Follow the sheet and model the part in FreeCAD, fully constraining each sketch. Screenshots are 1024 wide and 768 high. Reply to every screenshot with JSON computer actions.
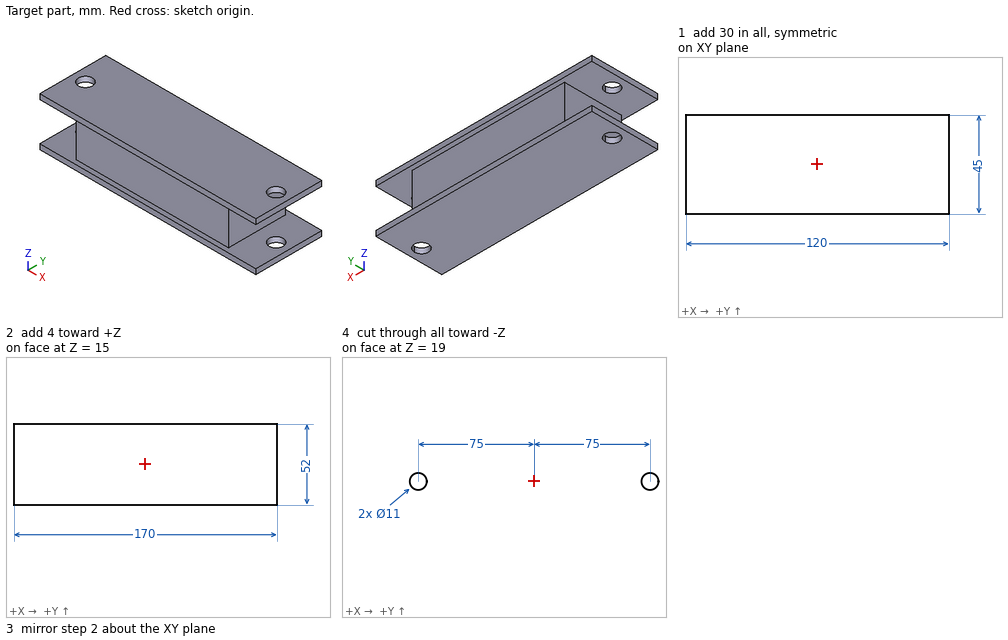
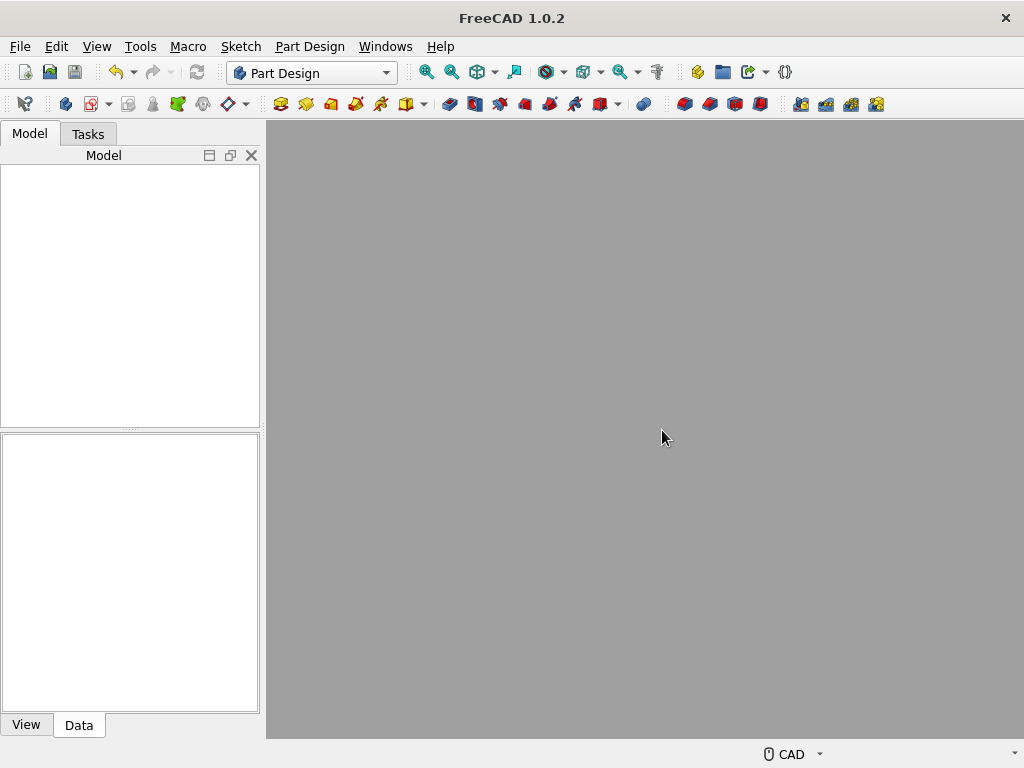
{"action": "left_click", "coordinate": [25, 72]}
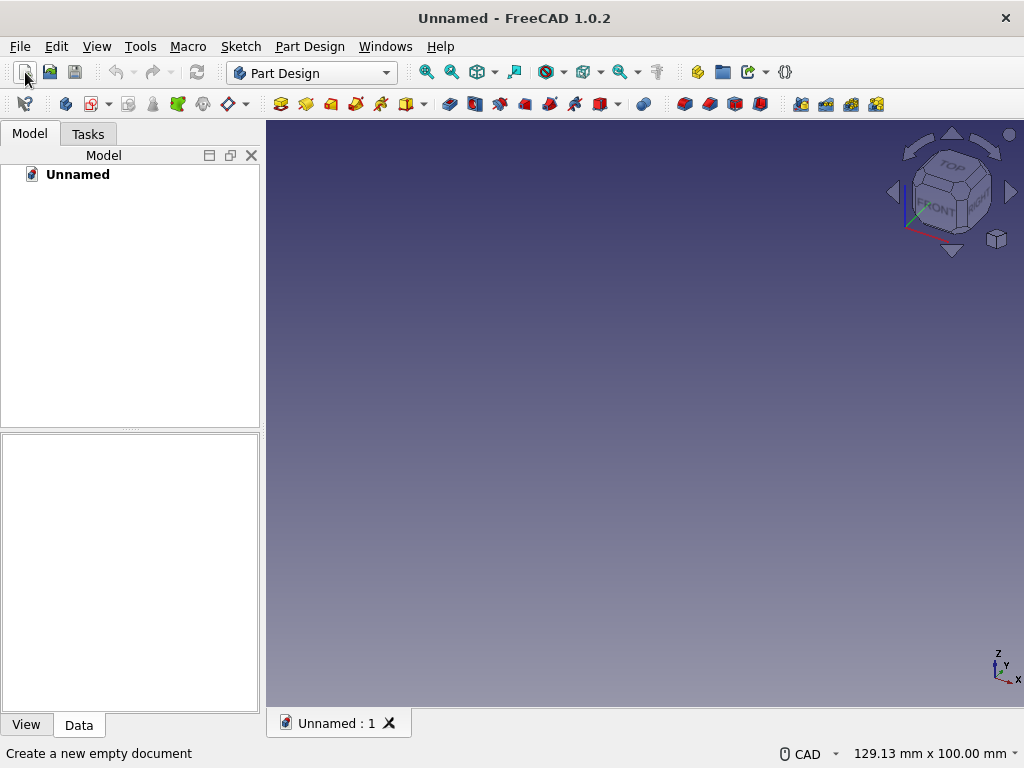
{"action": "left_click", "coordinate": [90, 104]}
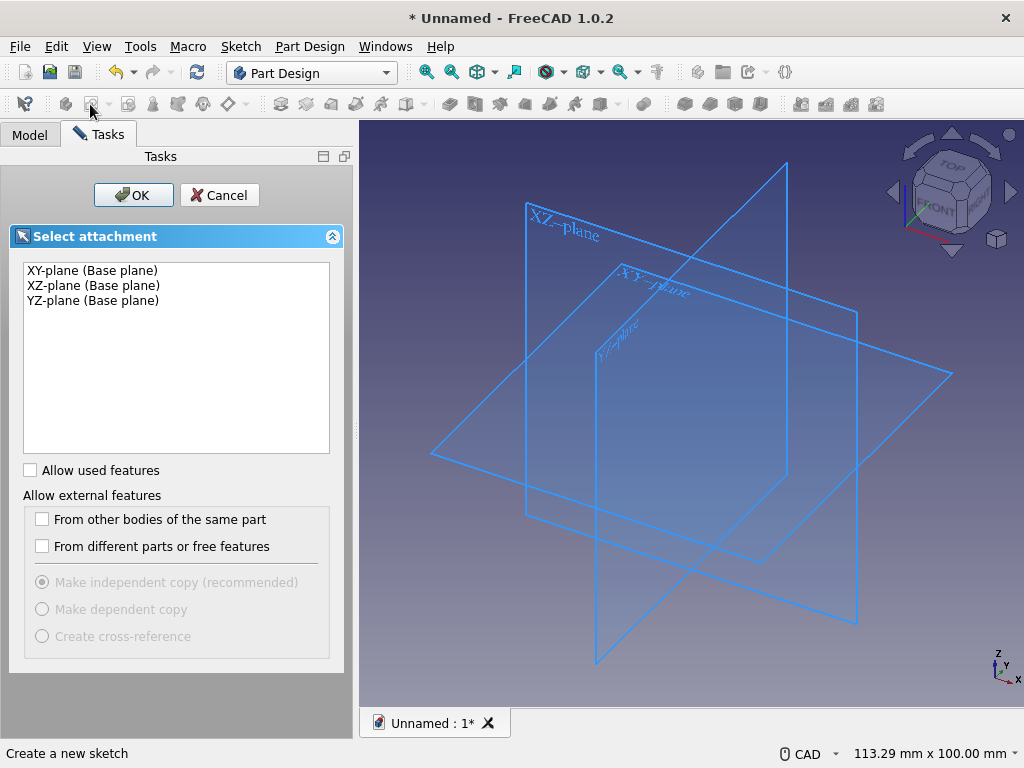
{"action": "left_click", "coordinate": [84, 270]}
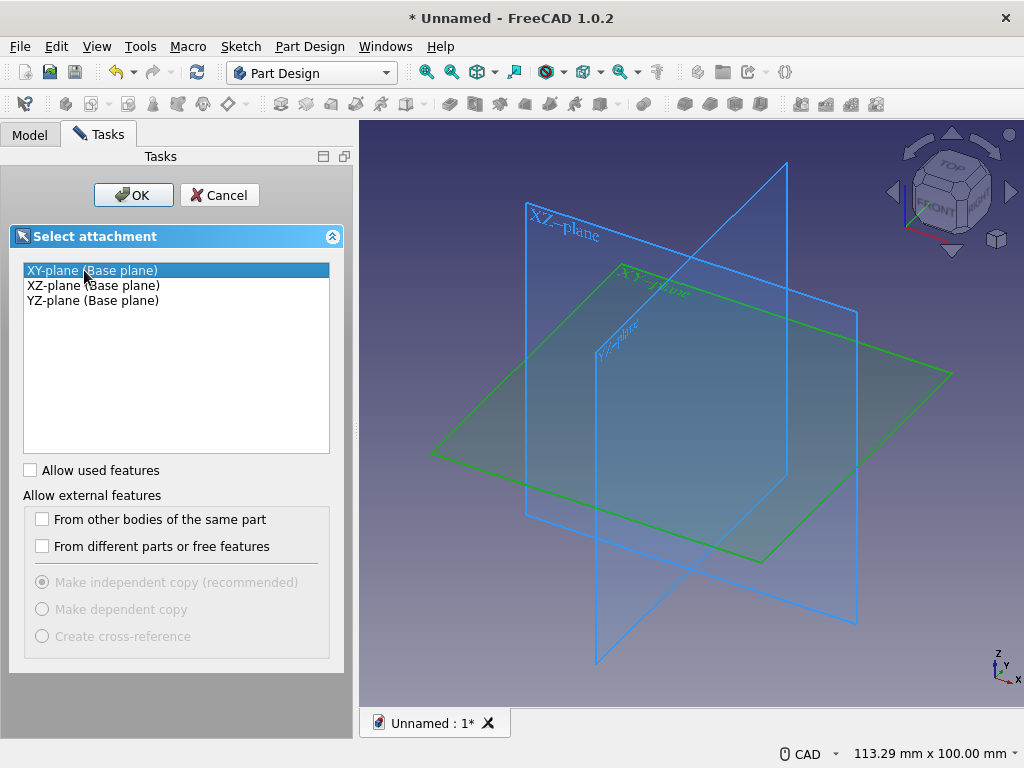
{"action": "left_click", "coordinate": [134, 195]}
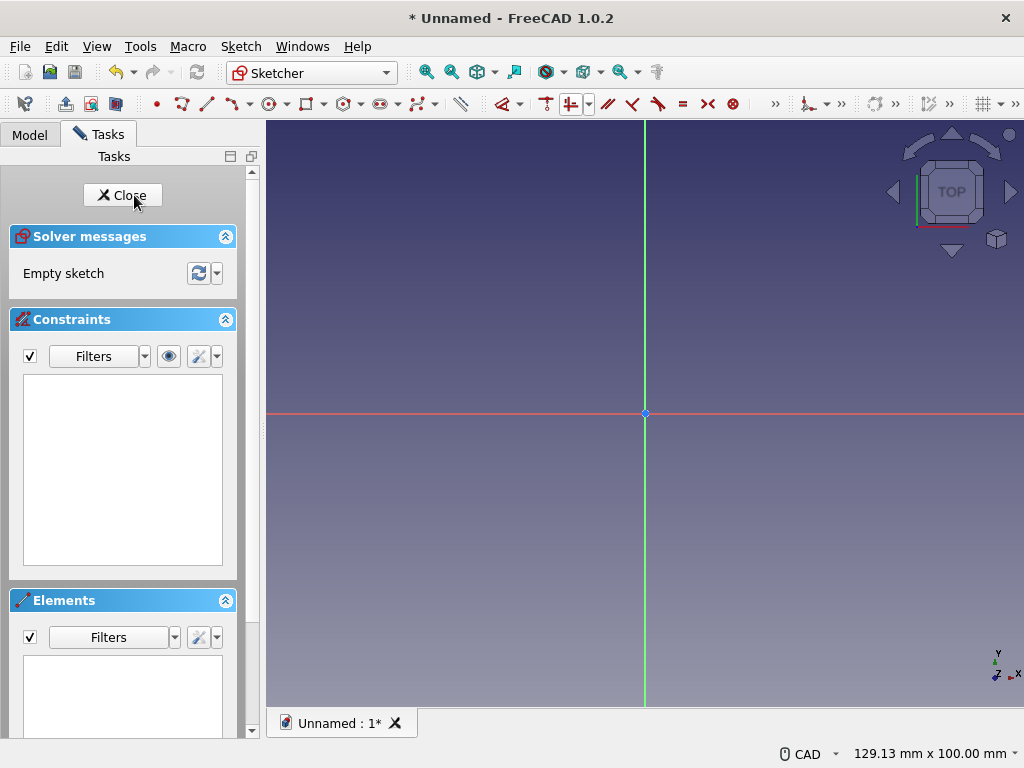
{"action": "scroll", "coordinate": [493, 414], "scroll_direction": "down", "scroll_amount": 3}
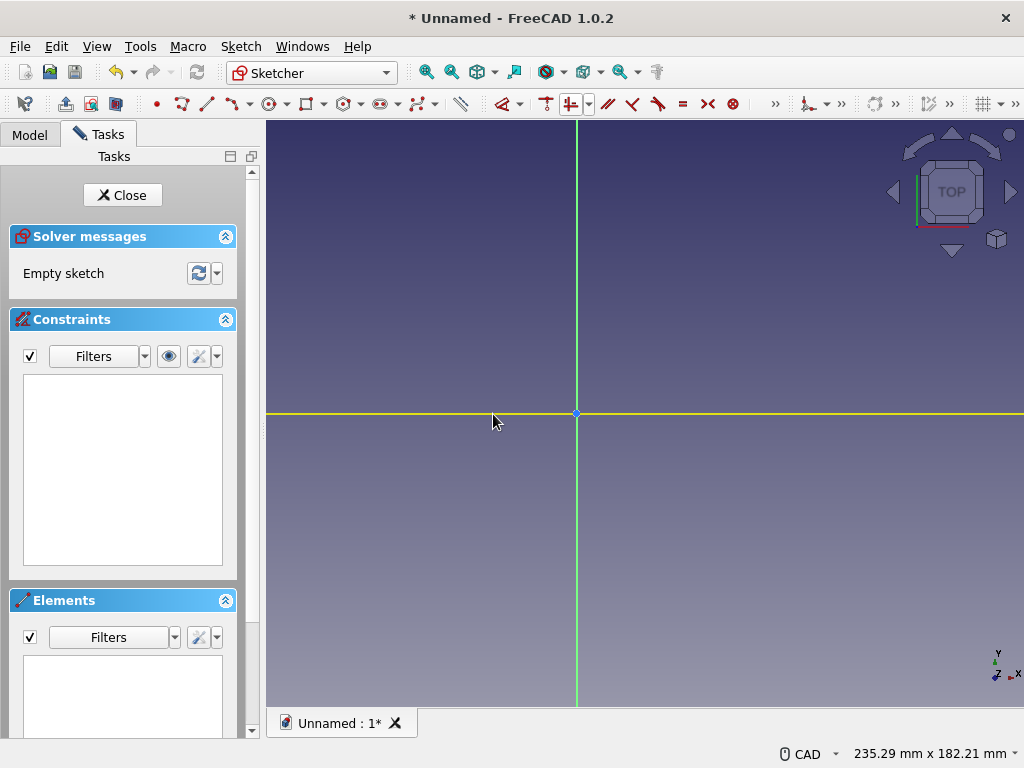
{"action": "left_click", "coordinate": [324, 104]}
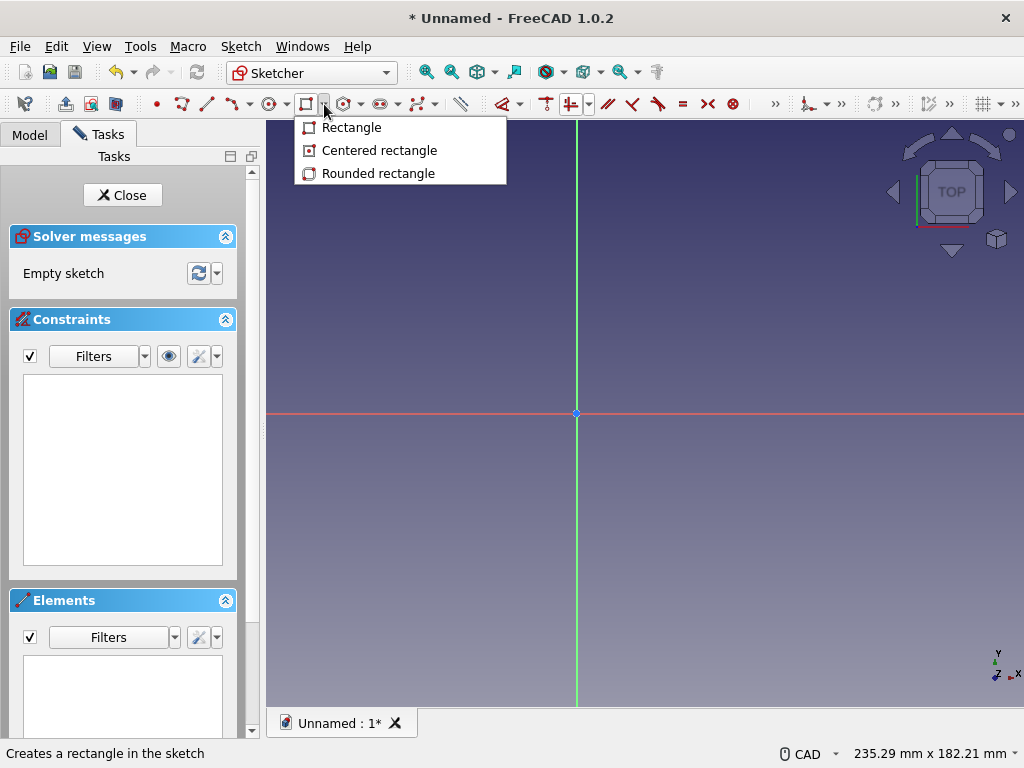
{"action": "left_click", "coordinate": [400, 150]}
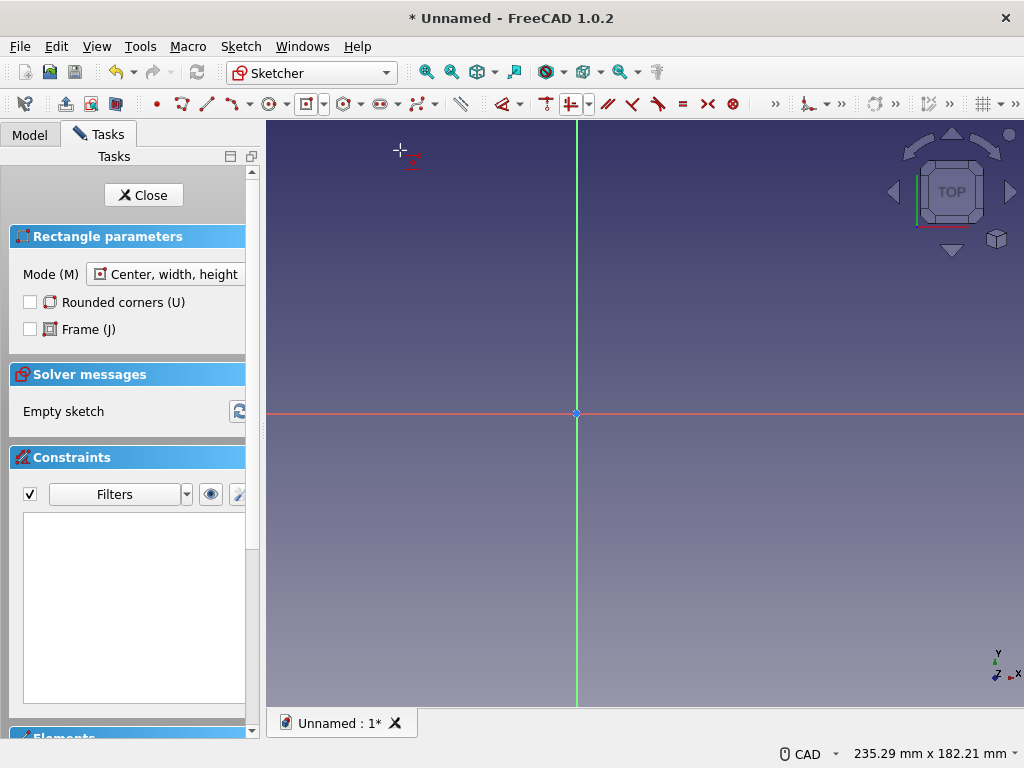
{"action": "left_click", "coordinate": [577, 414]}
{"action": "mouse_move", "coordinate": [770, 341]}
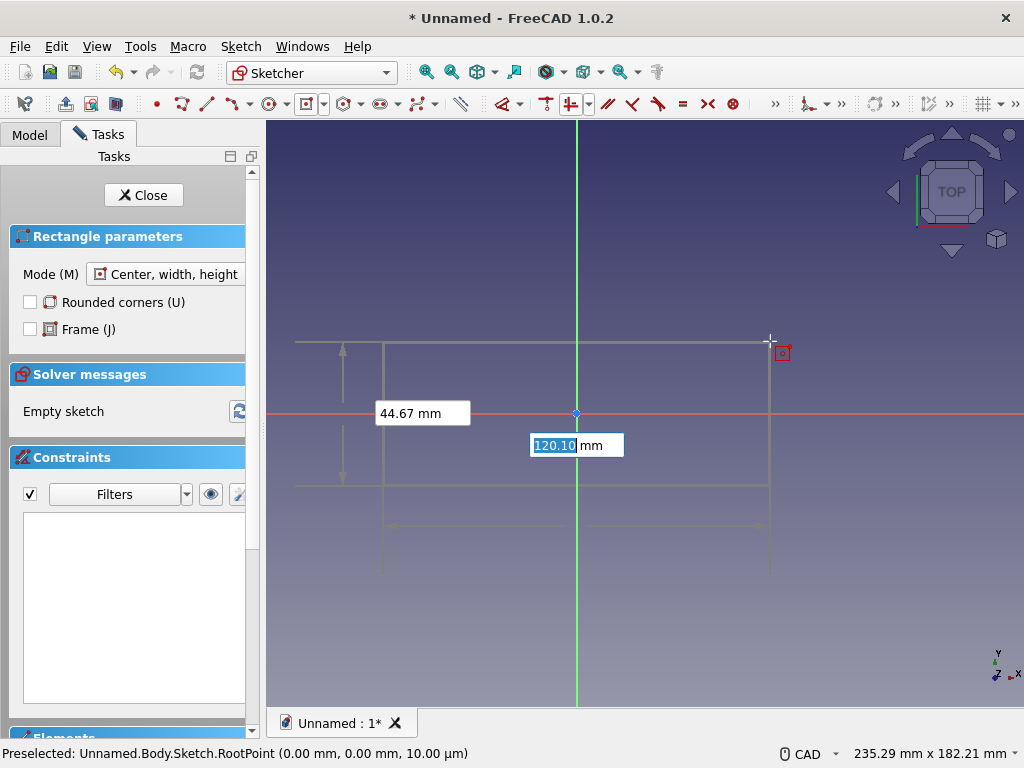
{"action": "type", "text": "120"}
{"action": "key", "text": "Tab"}
{"action": "type", "text": "45"}
{"action": "key", "text": "Return"}
{"action": "key", "text": "Escape"}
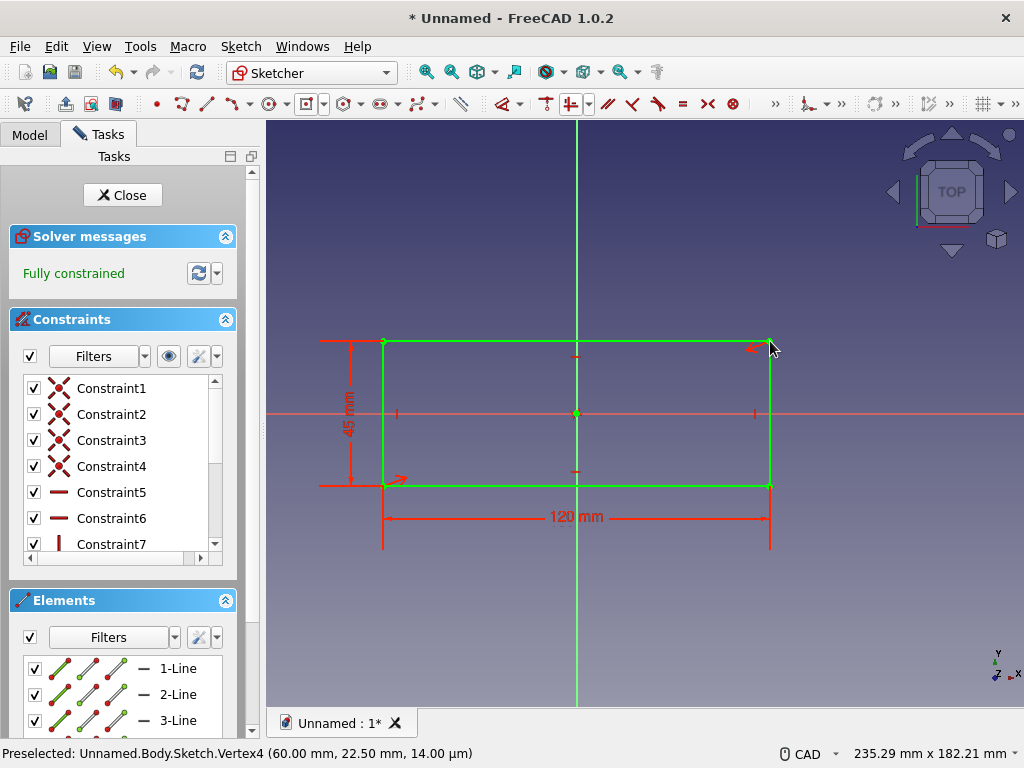
{"action": "left_click", "coordinate": [123, 195]}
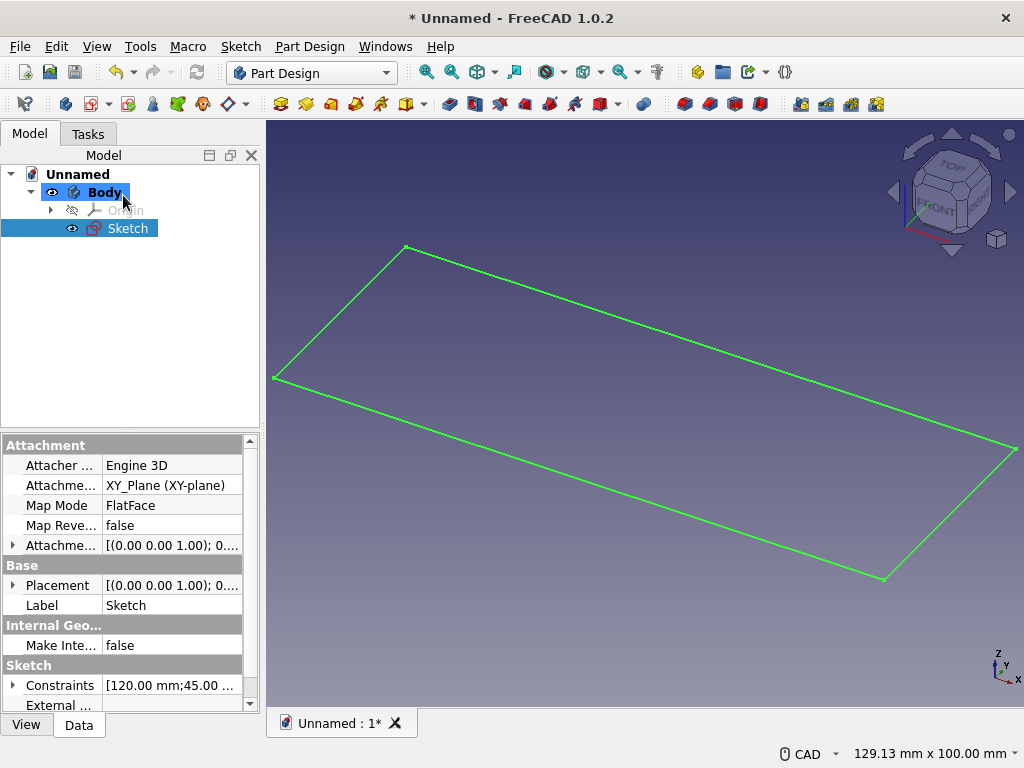
{"action": "left_click", "coordinate": [281, 104]}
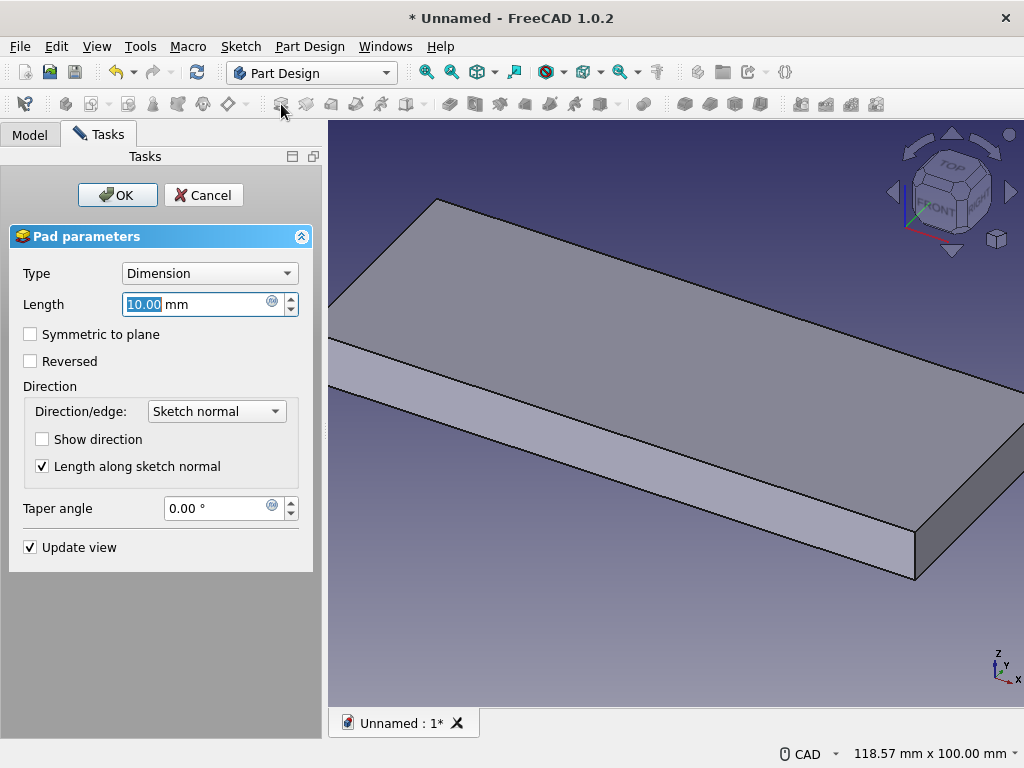
{"action": "type", "text": "30"}
{"action": "key", "text": "Tab"}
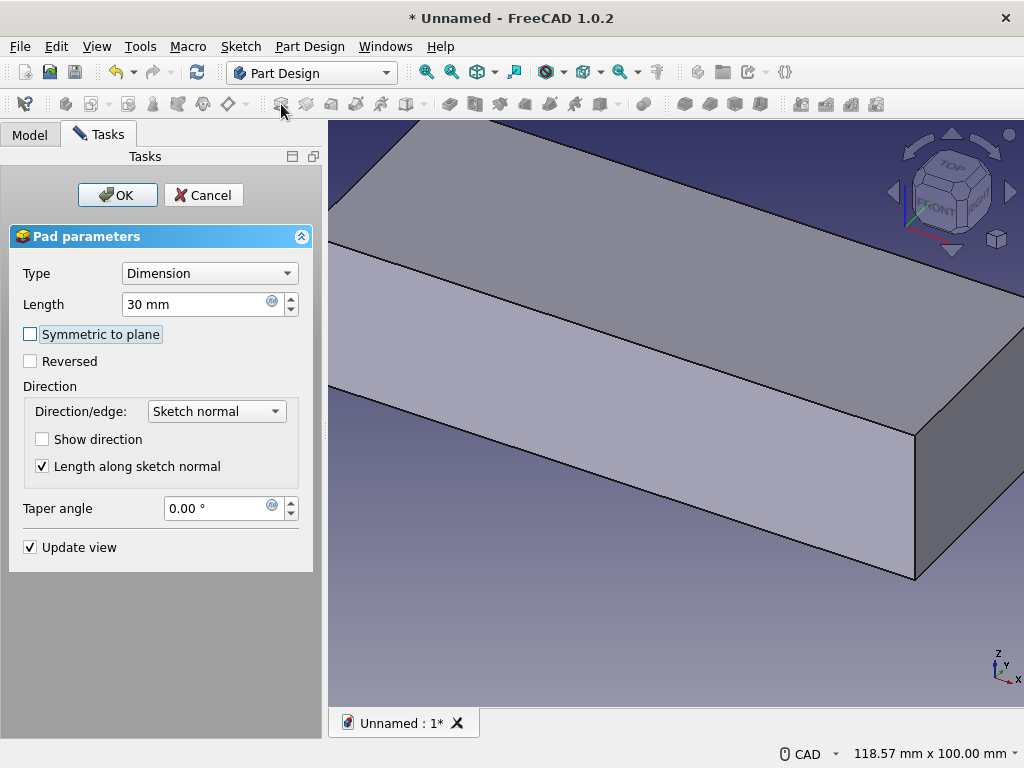
{"action": "left_click", "coordinate": [31, 334]}